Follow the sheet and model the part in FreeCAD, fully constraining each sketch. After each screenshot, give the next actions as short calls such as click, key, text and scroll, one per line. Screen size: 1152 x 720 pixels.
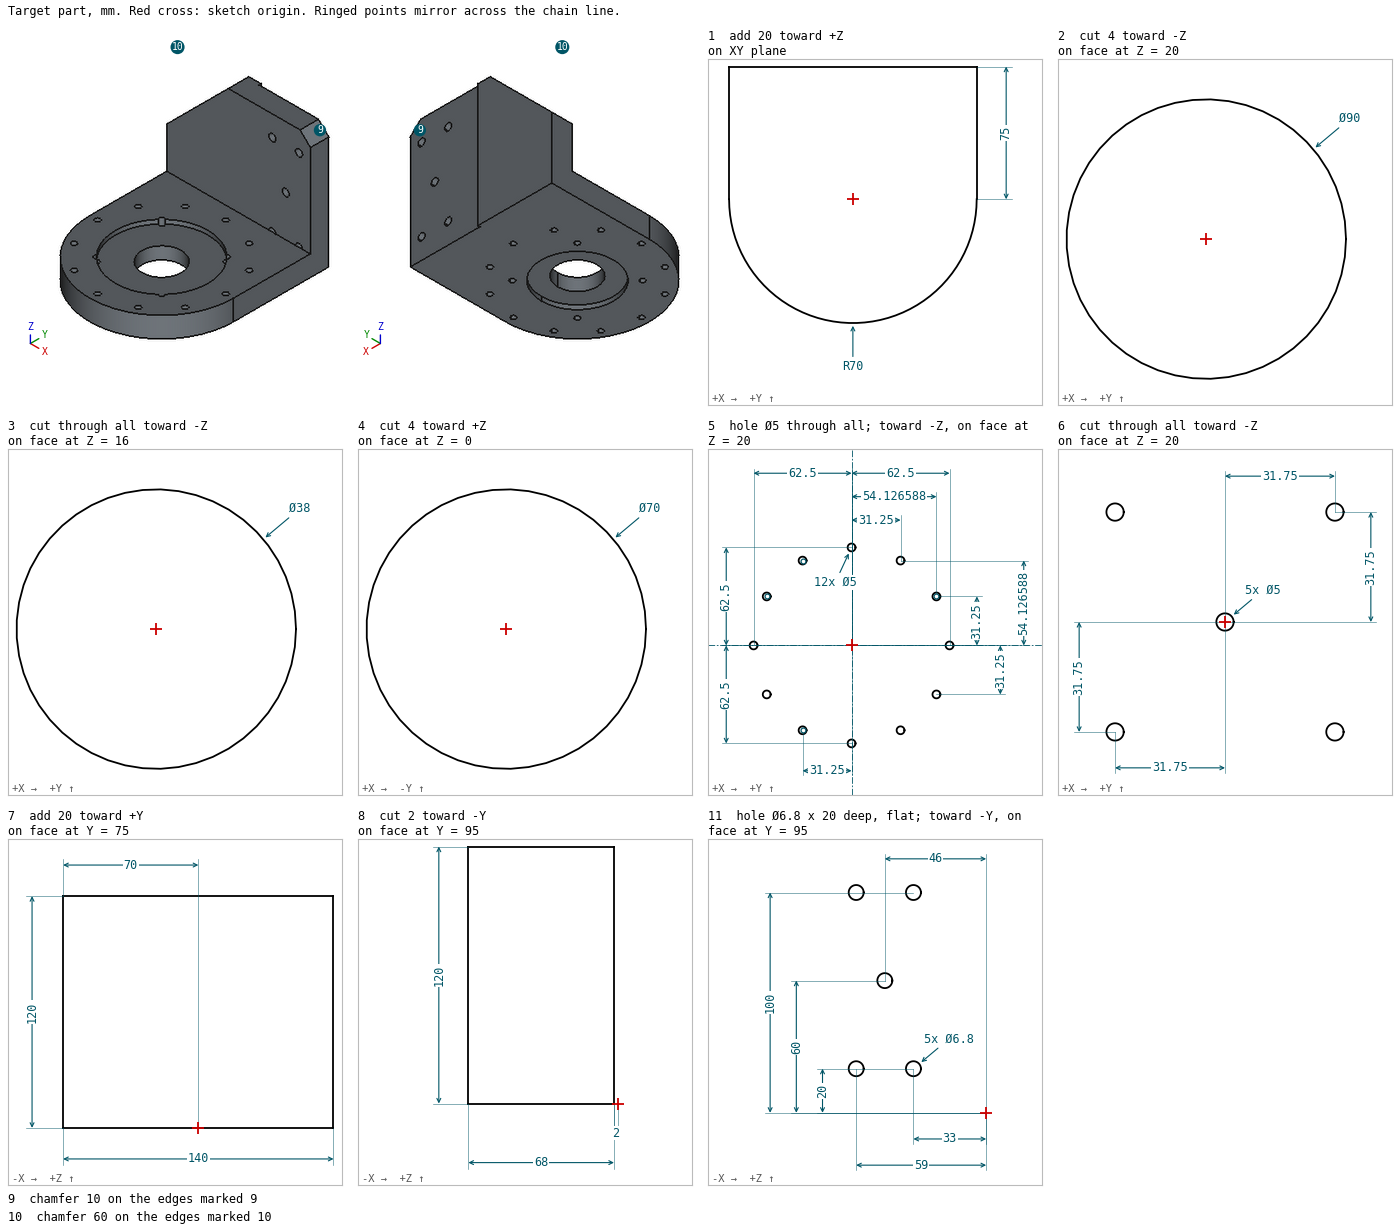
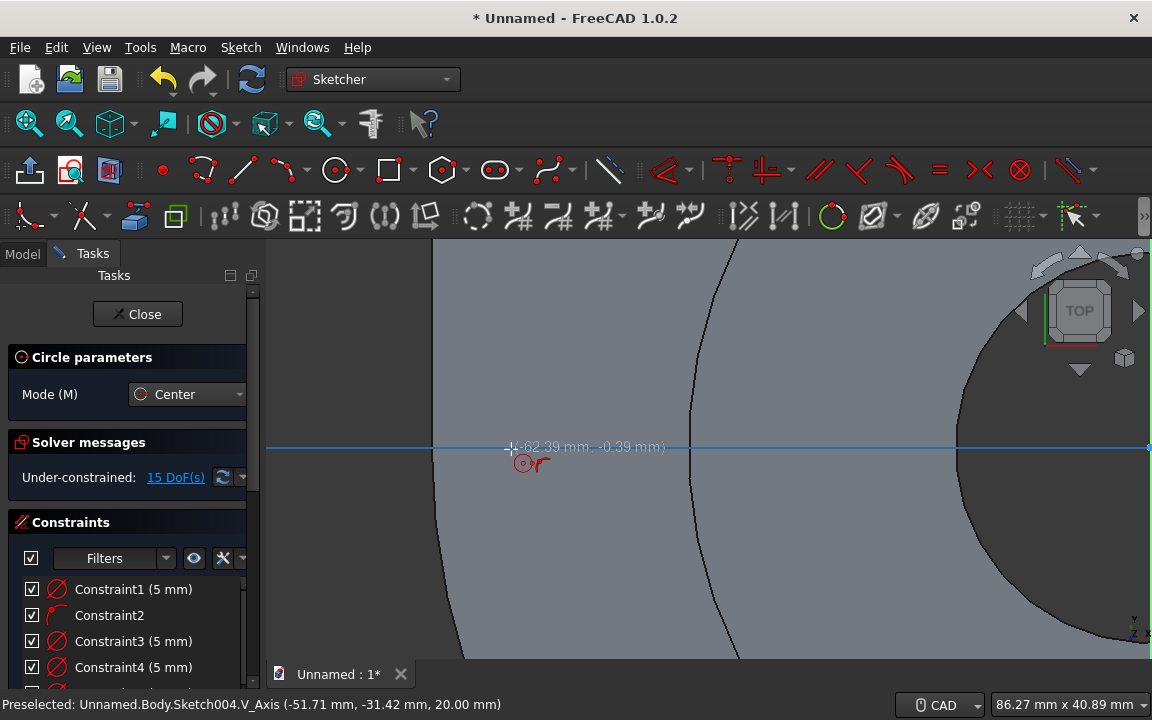
scroll(511, 449, down, 8)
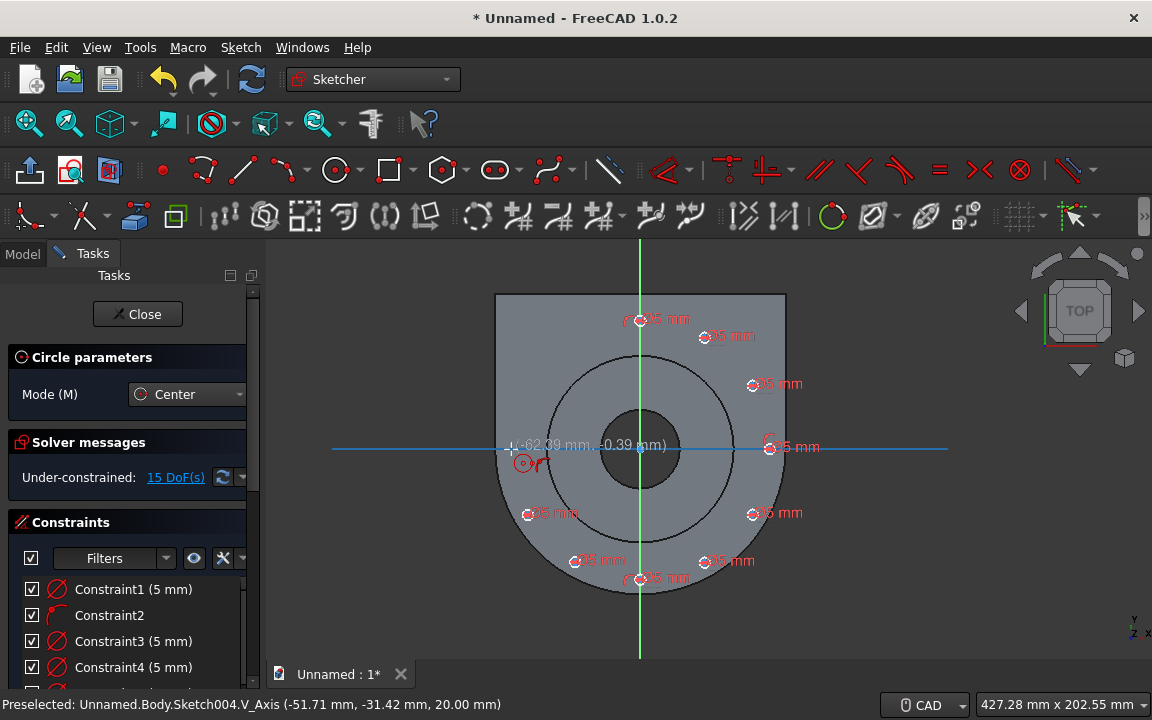
click(511, 449)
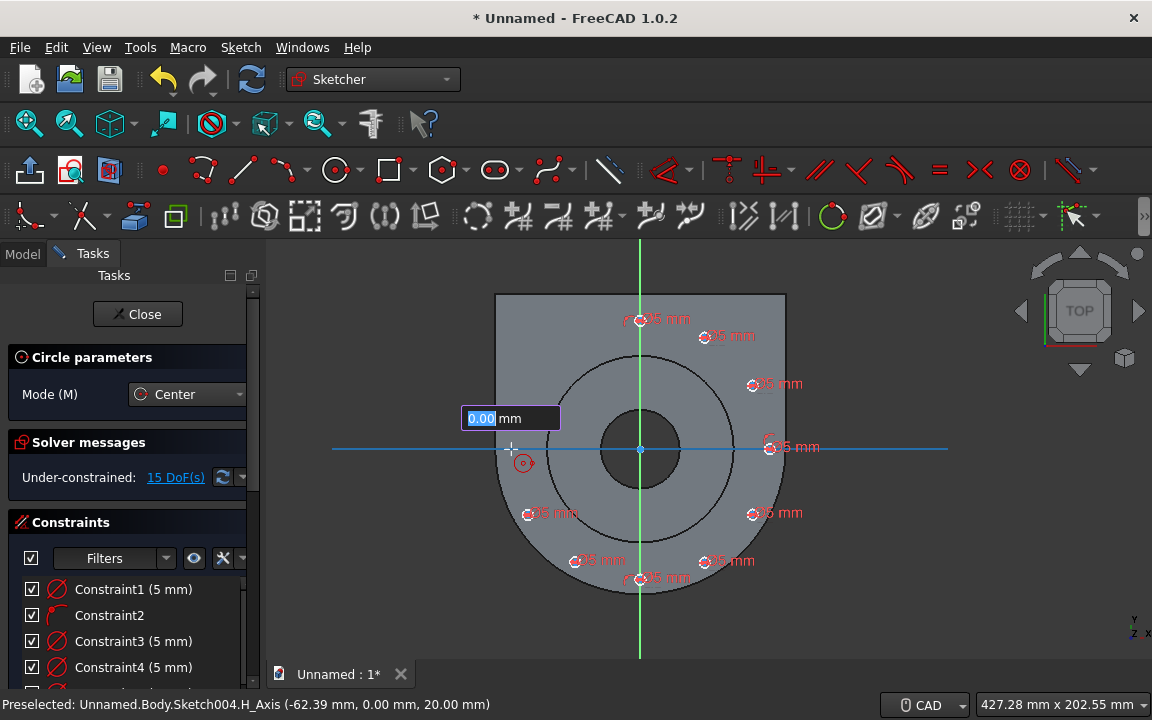
scroll(509, 454, up, 6)
move(508, 453)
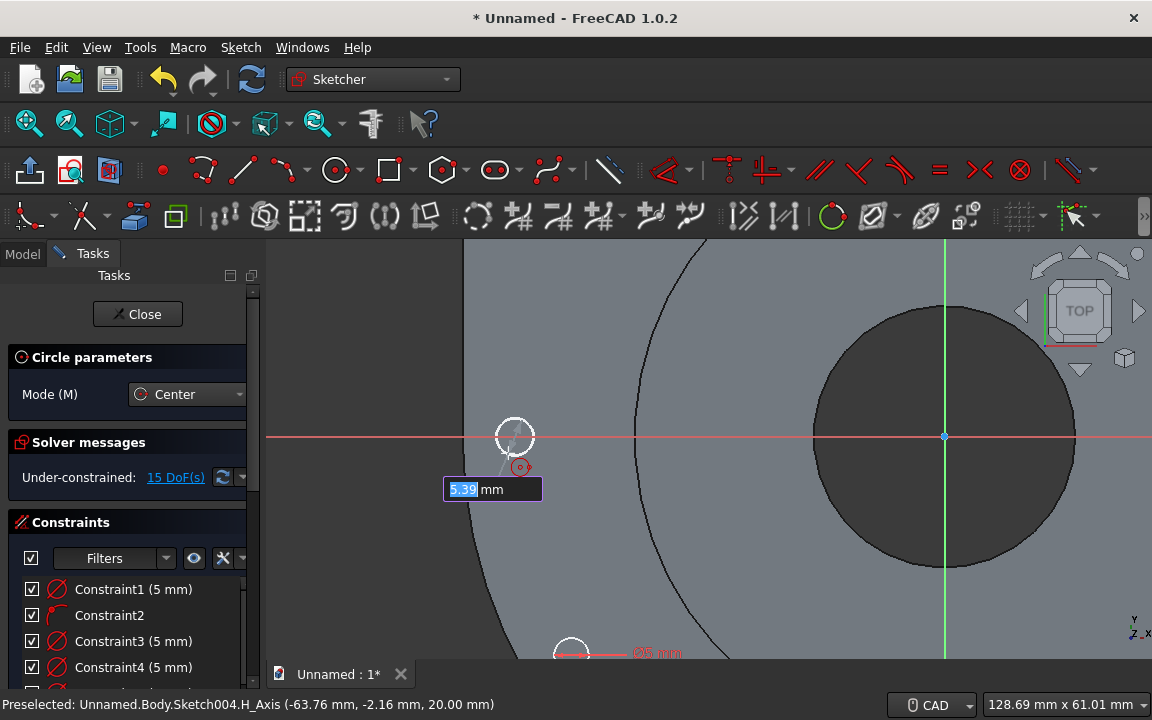
text(5)
key(Return)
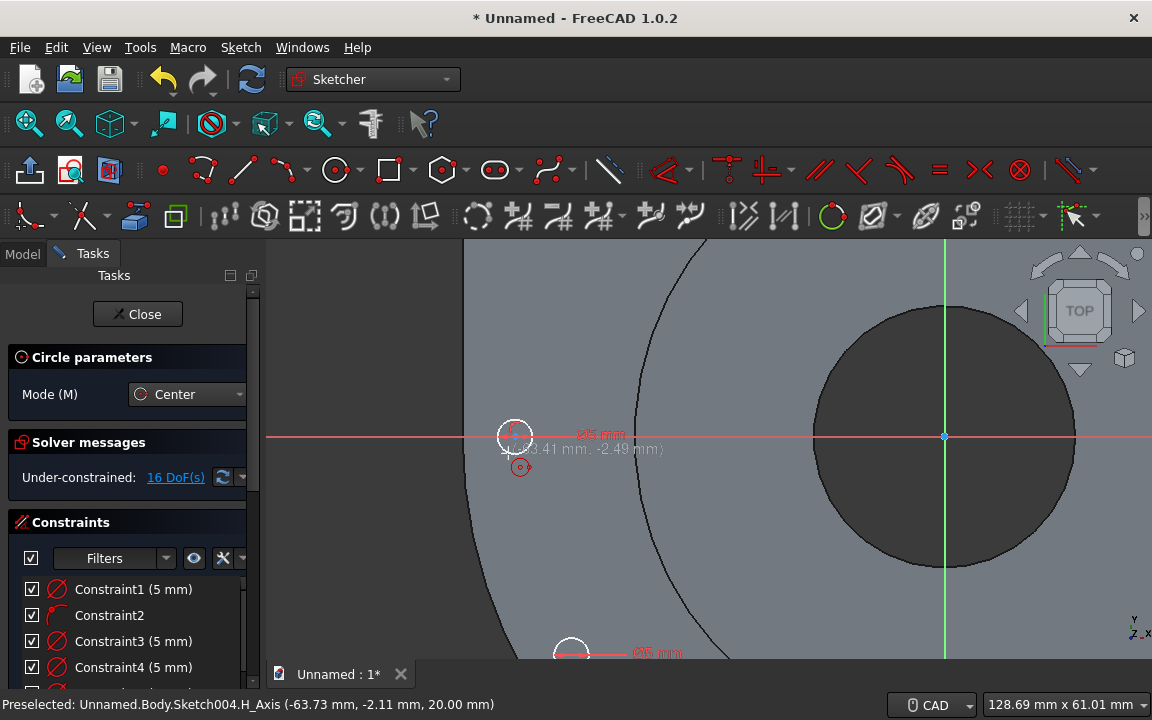
scroll(509, 454, down, 6)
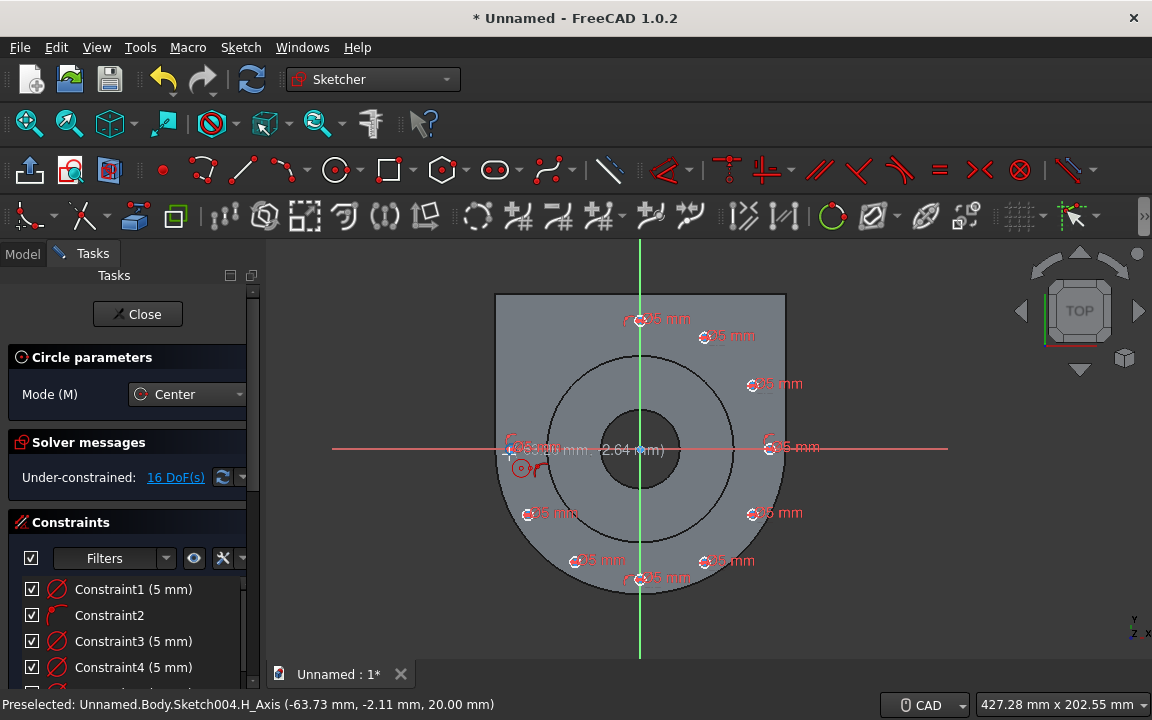
scroll(528, 384, up, 8)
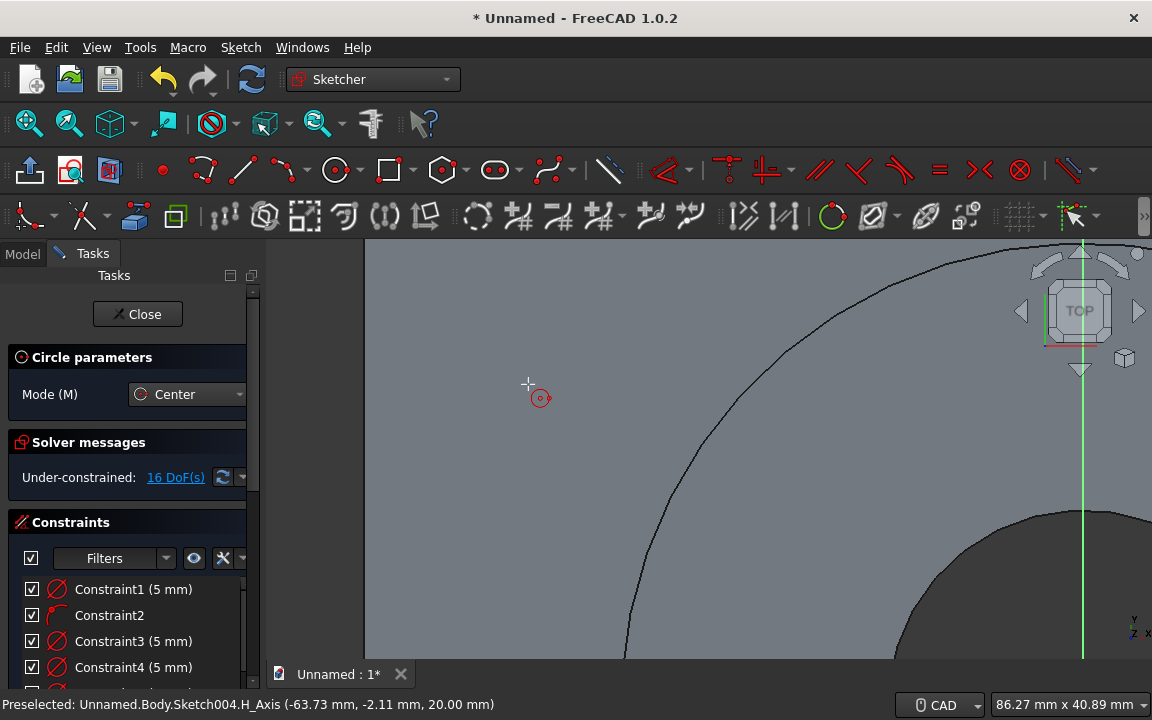
scroll(528, 384, down, 8)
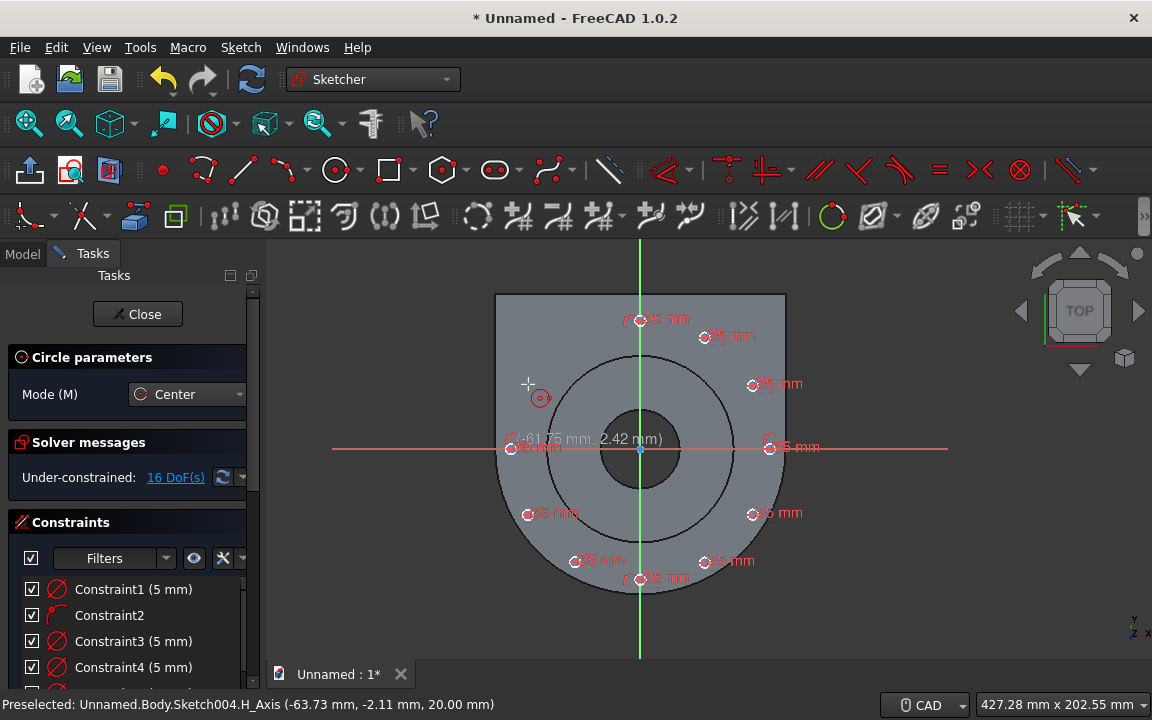
click(528, 384)
move(532, 381)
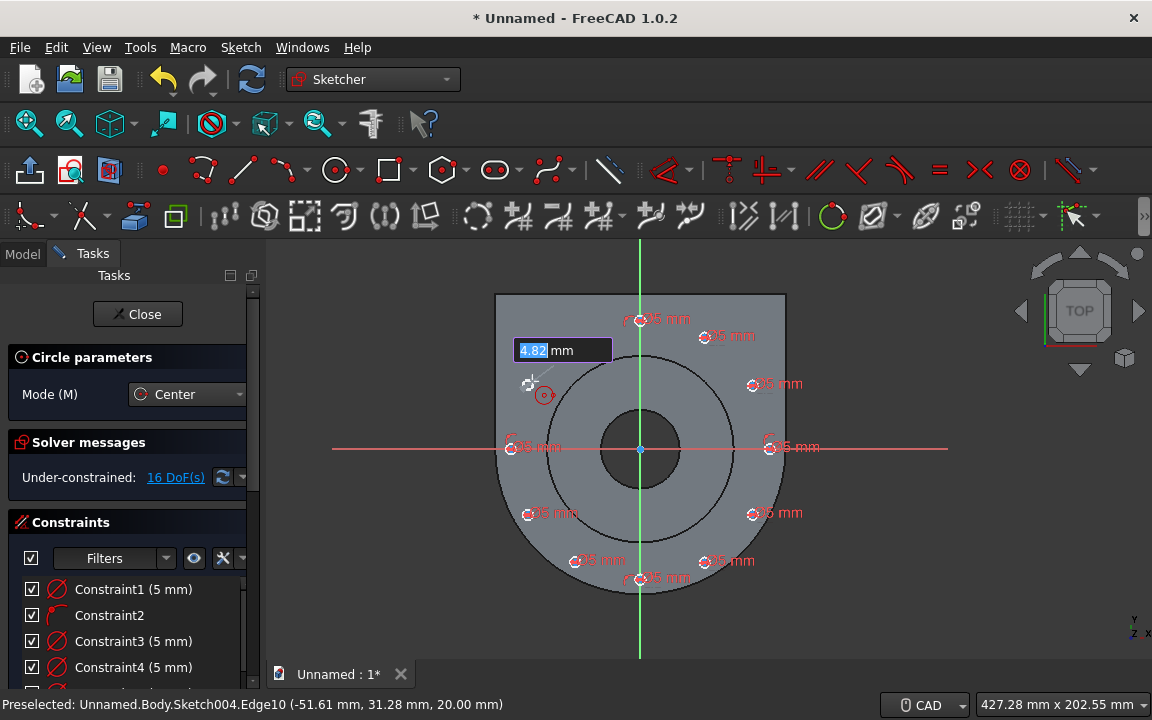
text(5)
key(Return)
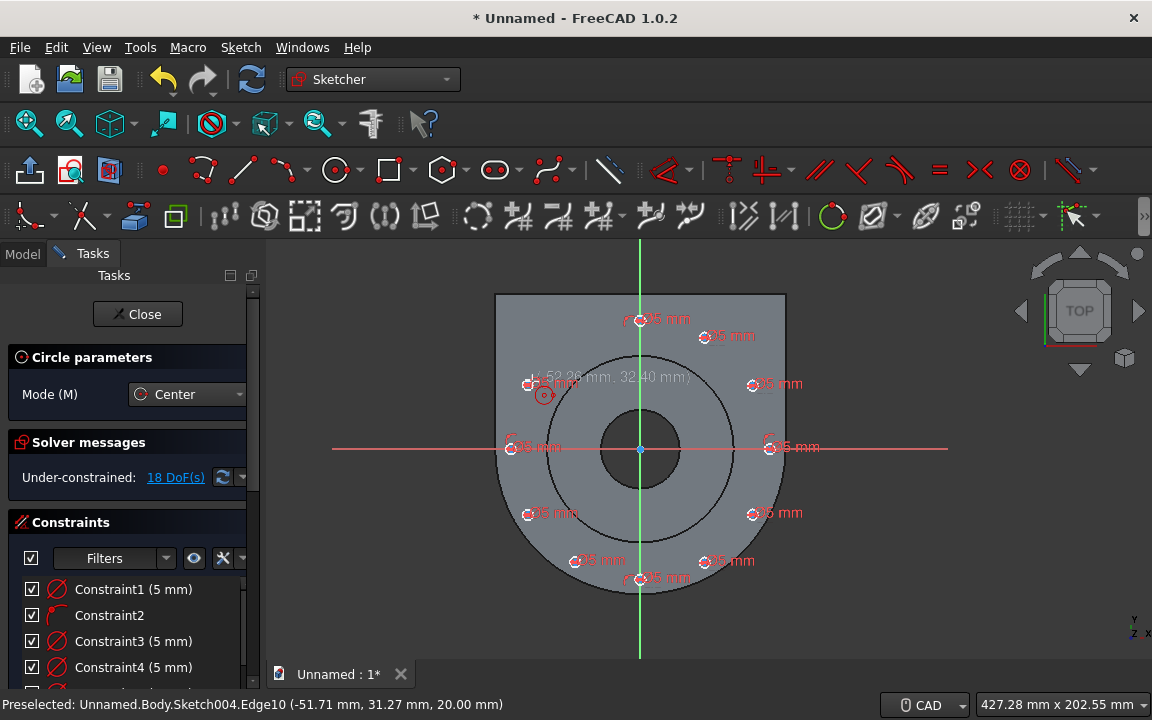
scroll(576, 337, up, 8)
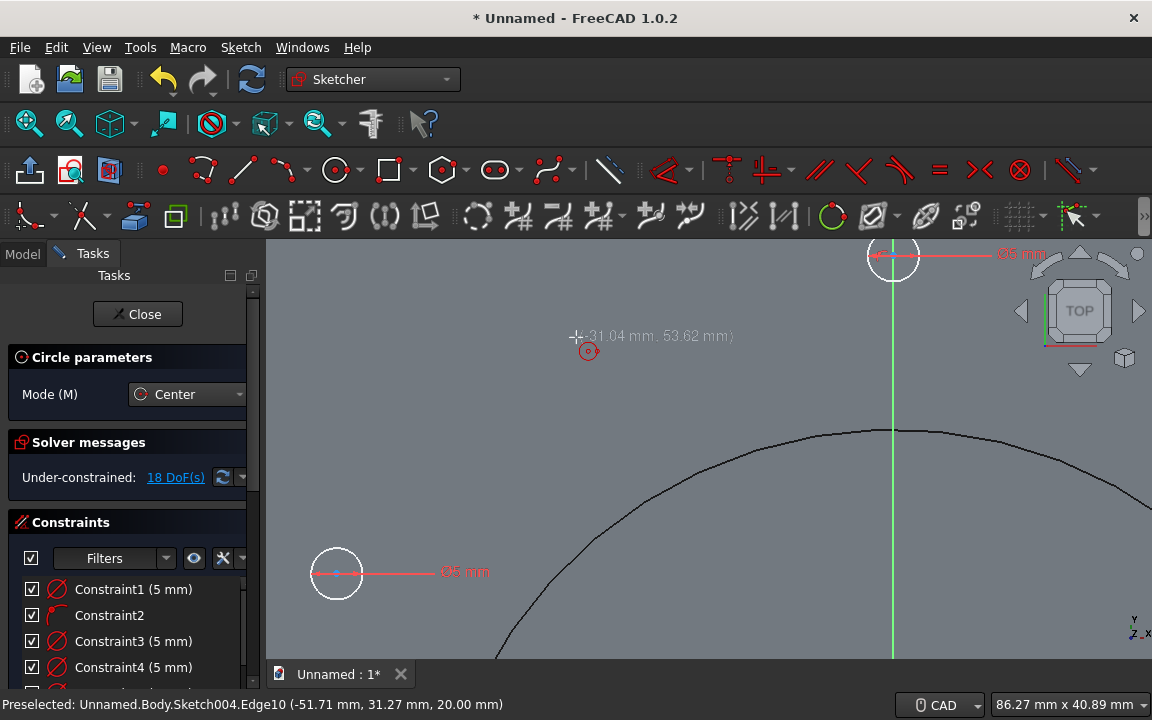
scroll(577, 337, down, 8)